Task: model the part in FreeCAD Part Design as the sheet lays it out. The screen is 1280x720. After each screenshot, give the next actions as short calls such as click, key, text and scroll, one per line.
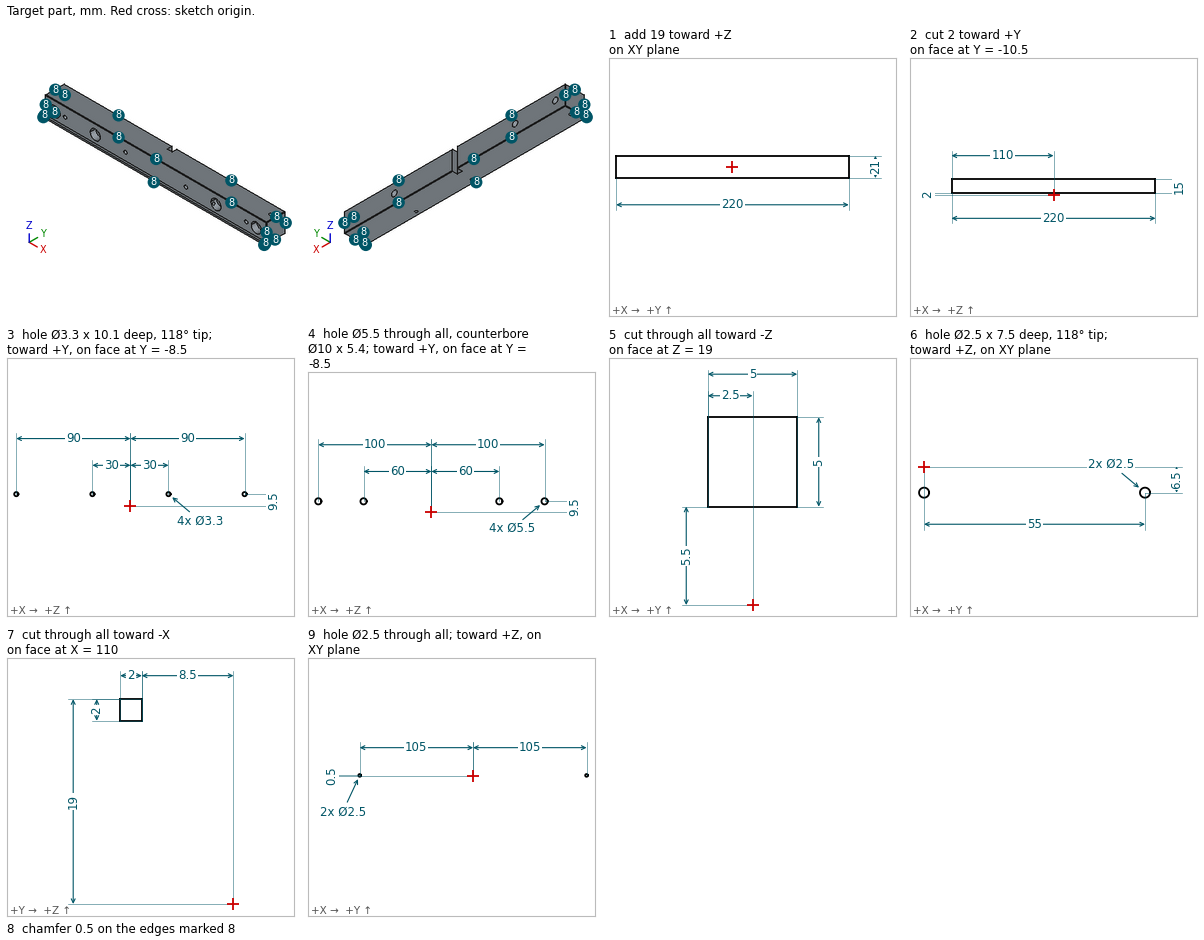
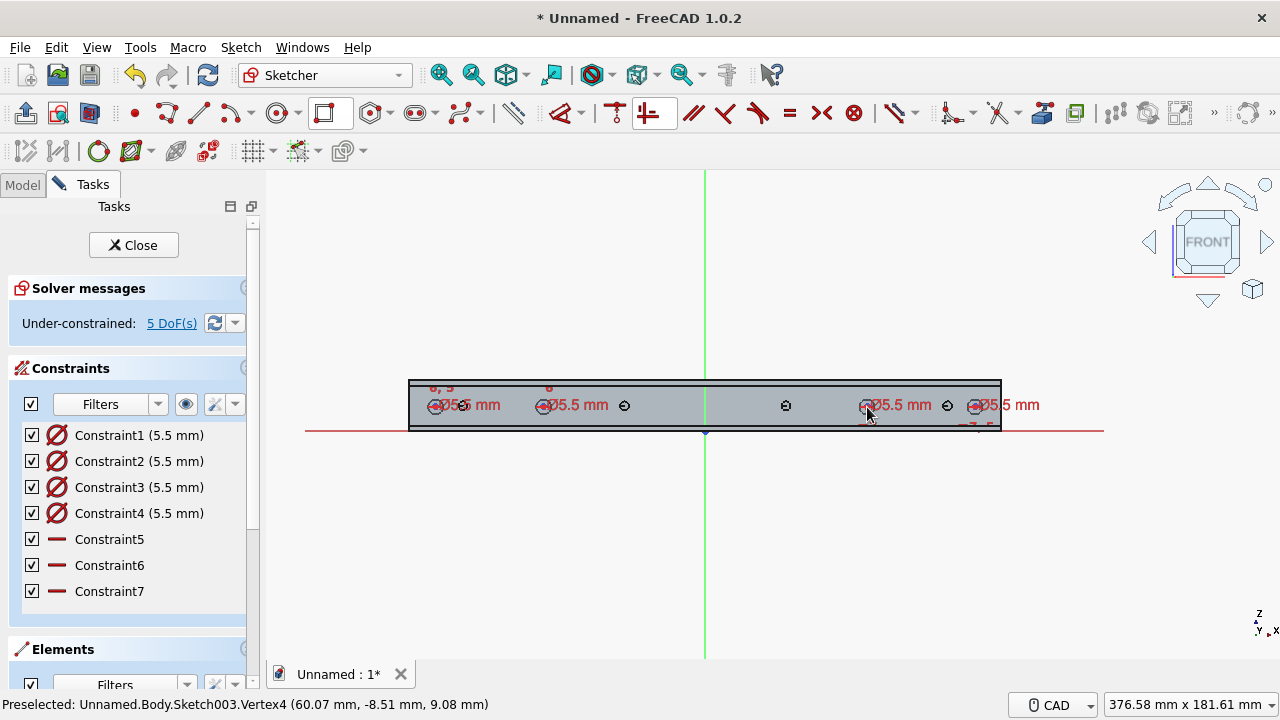
click(560, 114)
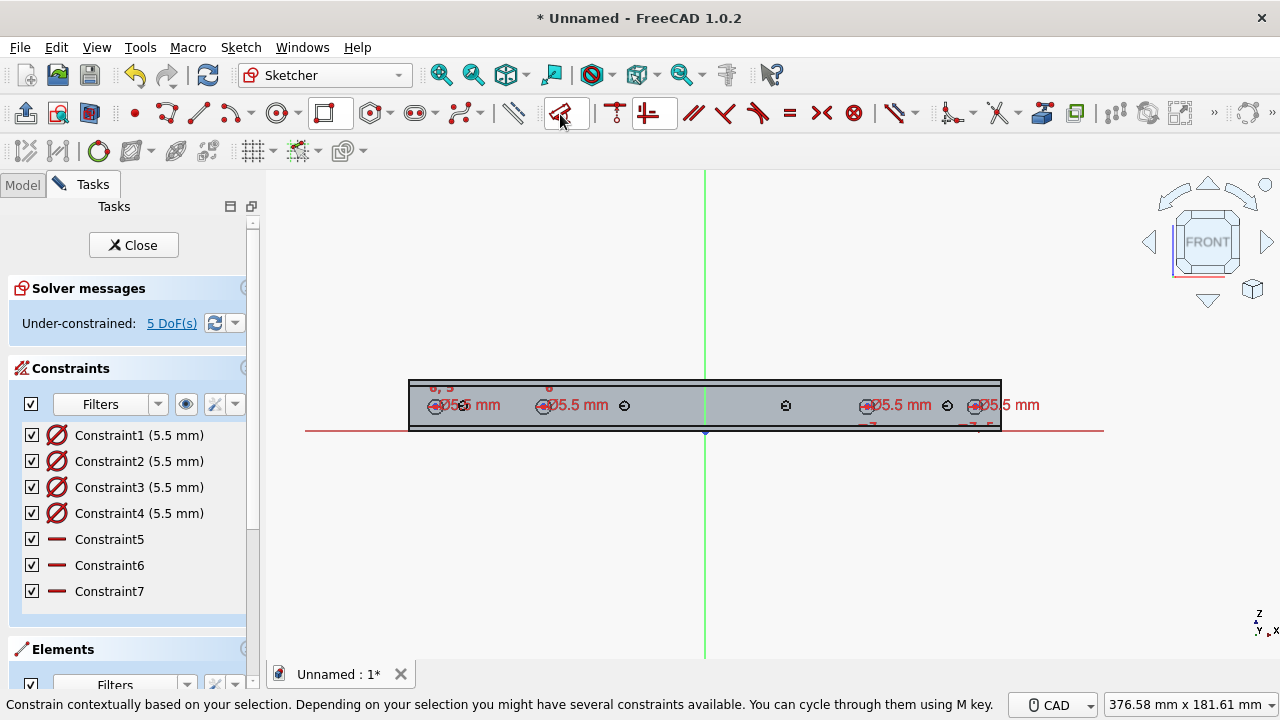
click(544, 407)
click(624, 465)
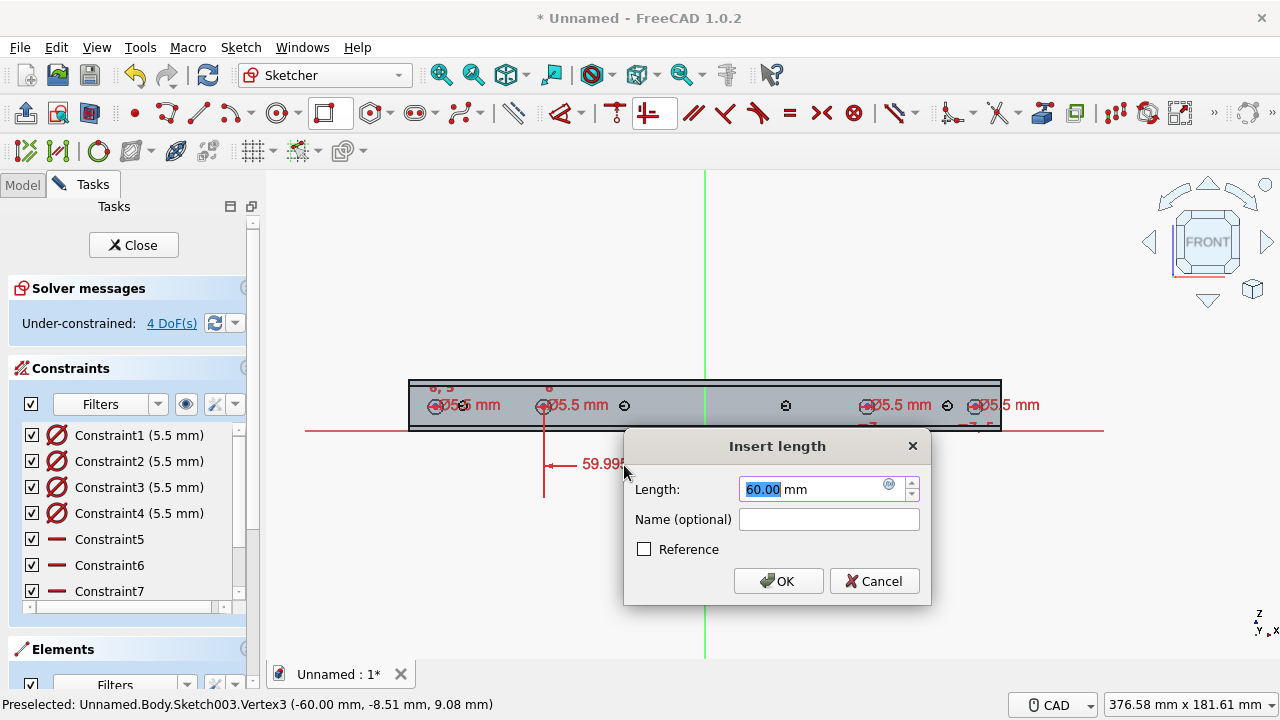
text(60)
key(Return)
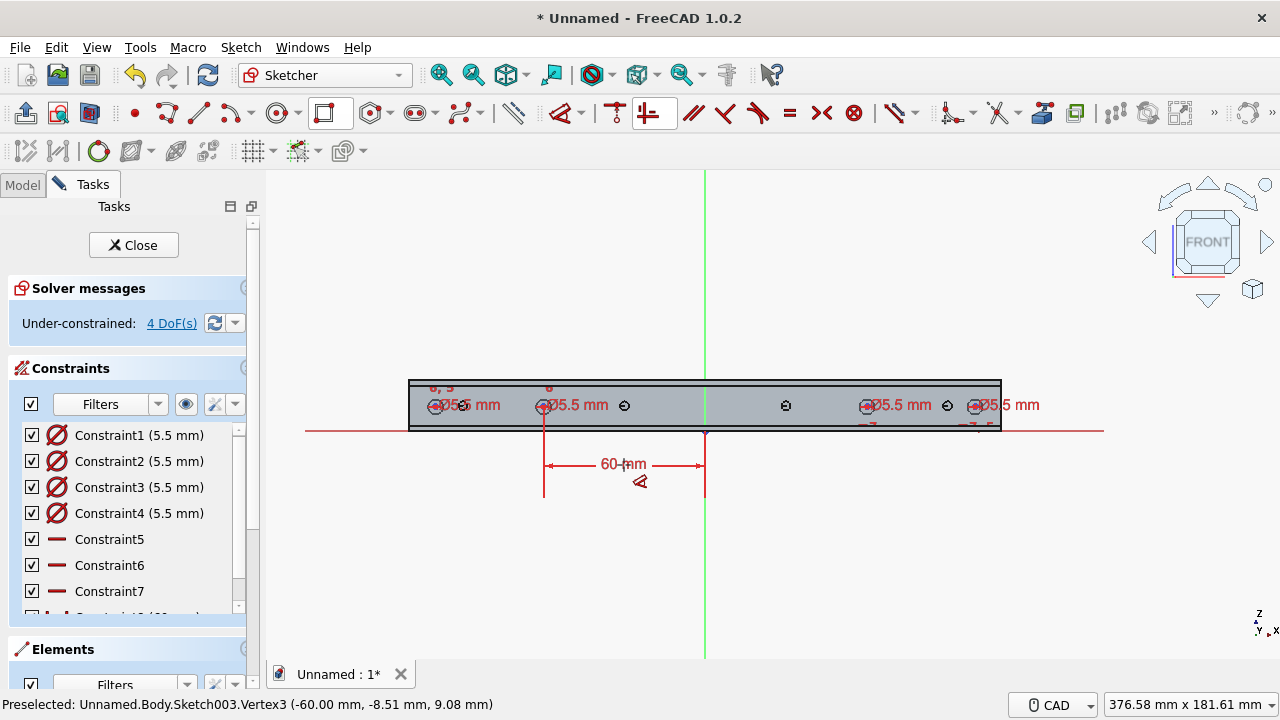
click(867, 407)
click(786, 465)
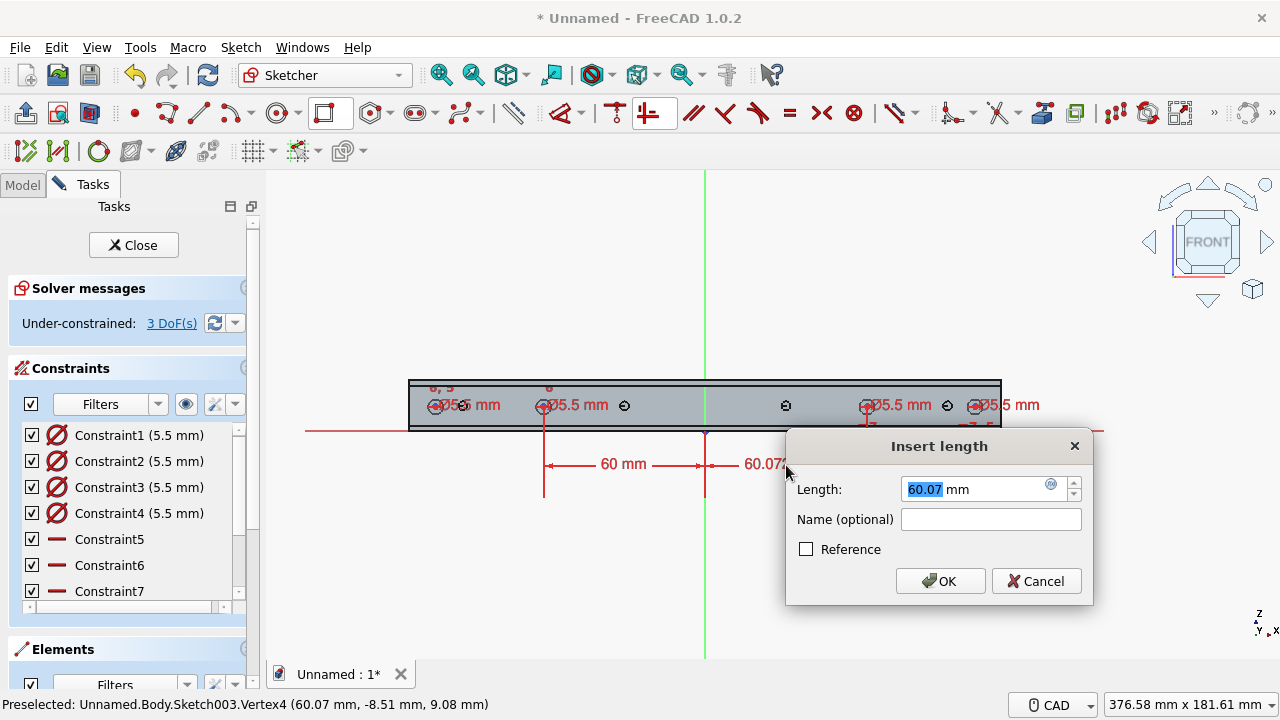
text(60)
key(Return)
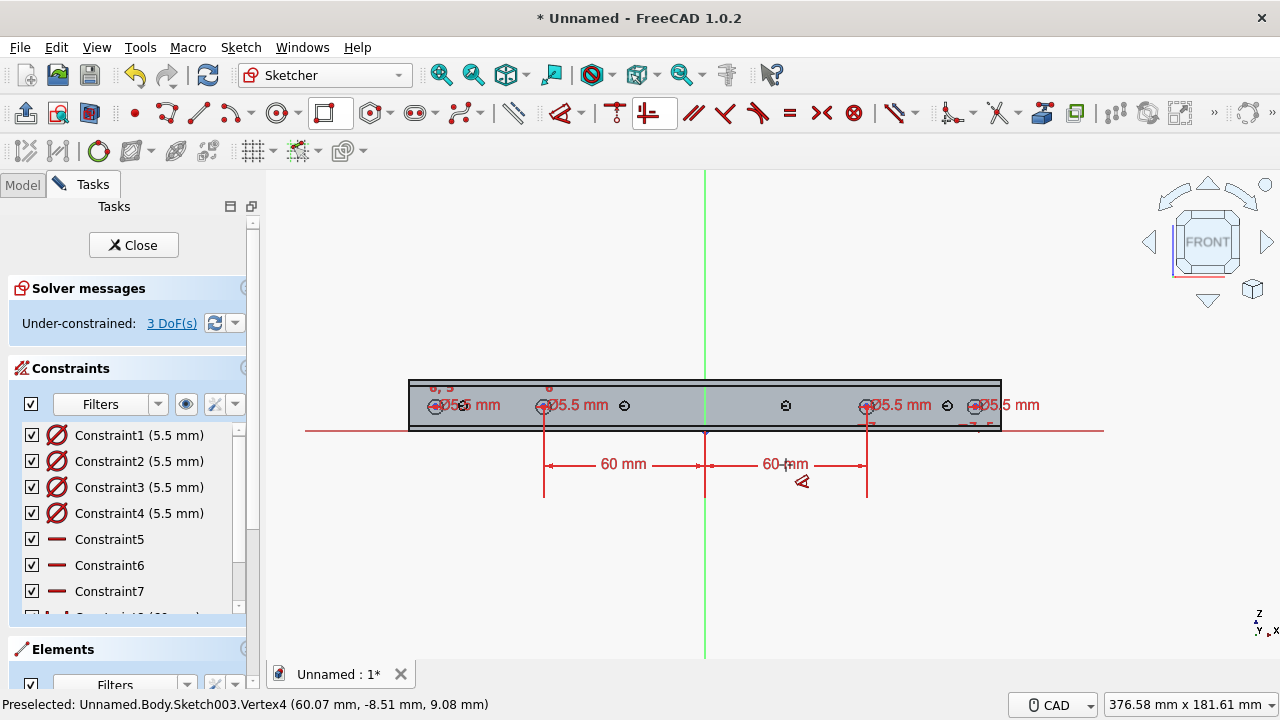
click(975, 407)
click(902, 465)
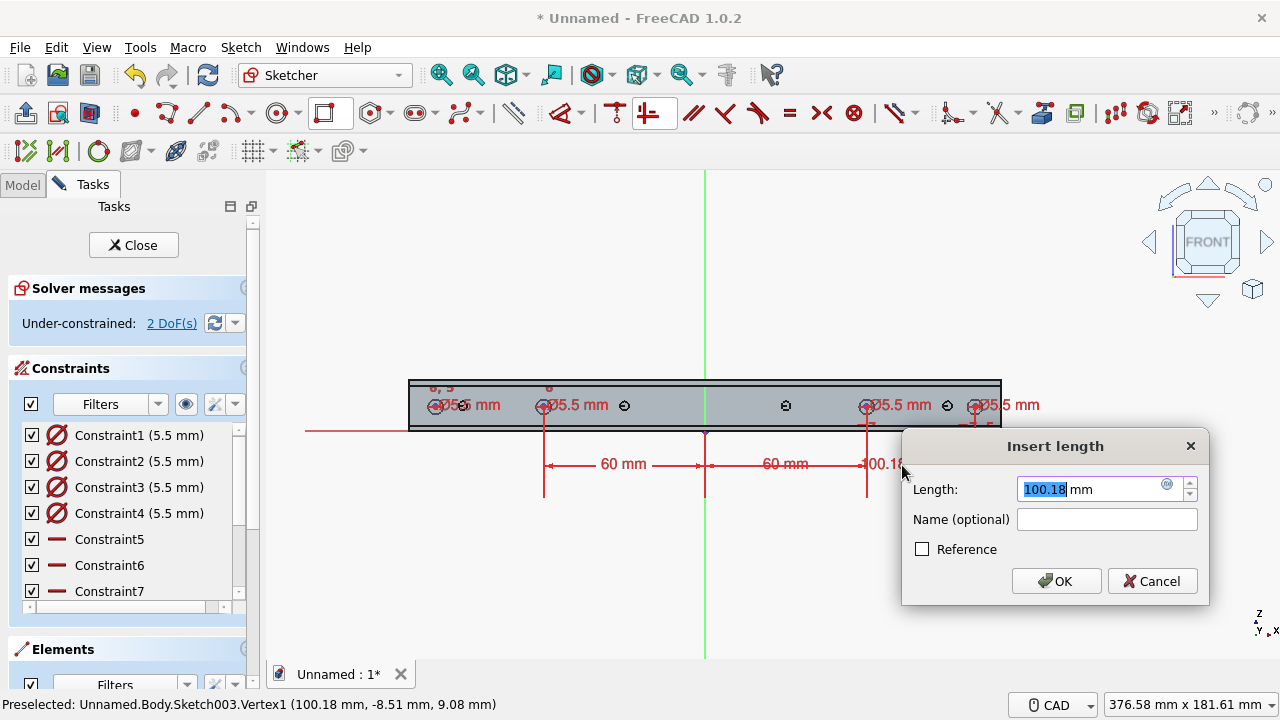
text(100)
key(Return)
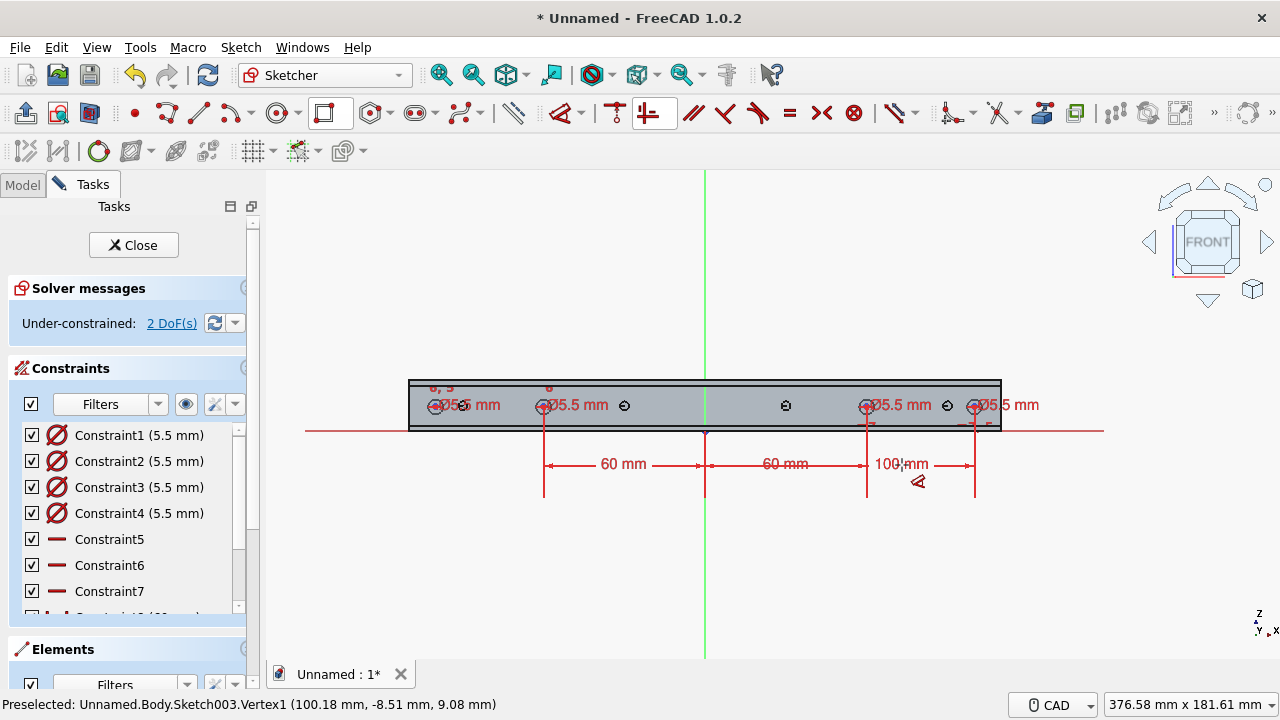
scroll(975, 407, up, 3)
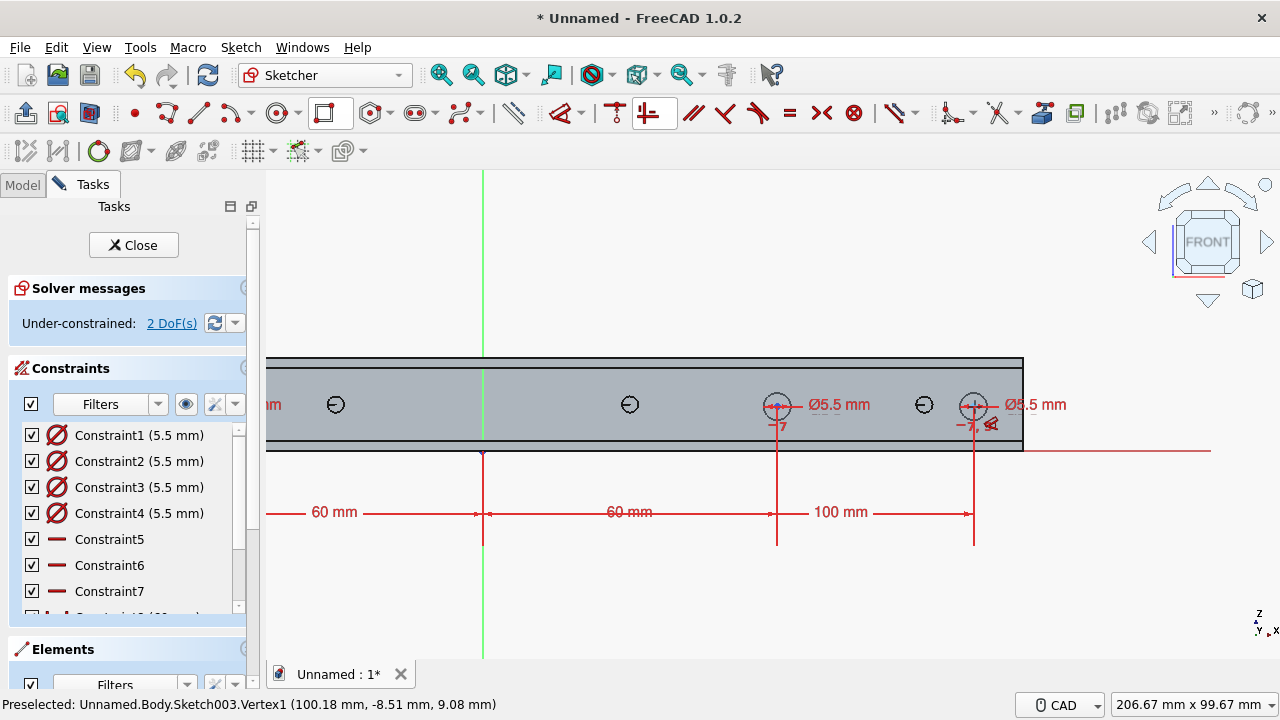
click(974, 407)
click(1008, 429)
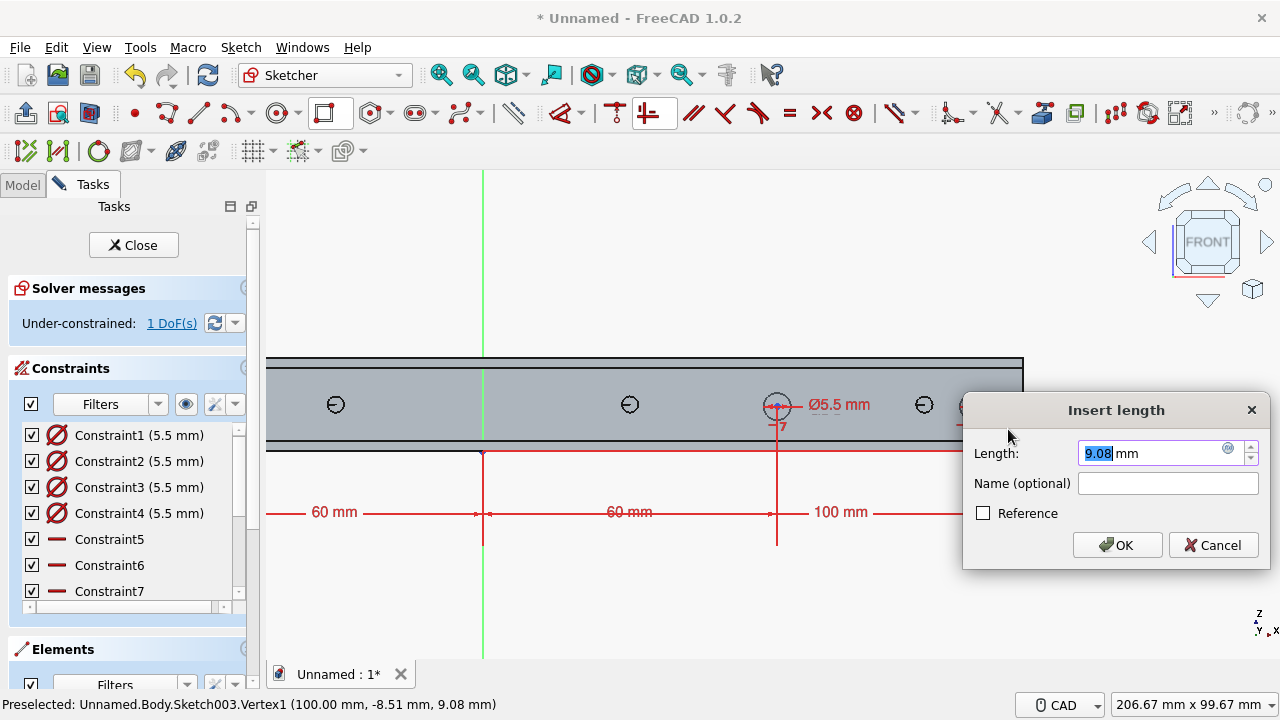
text(9.5)
key(Return)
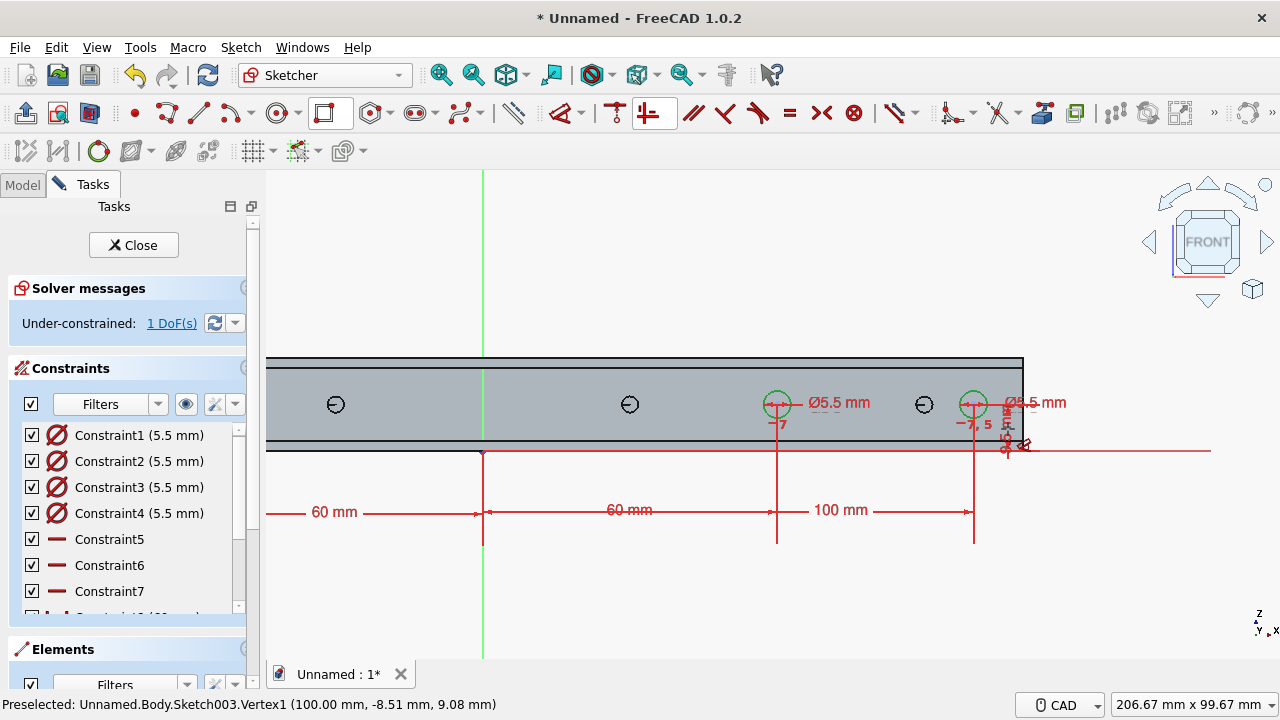
scroll(974, 406, down, 3)